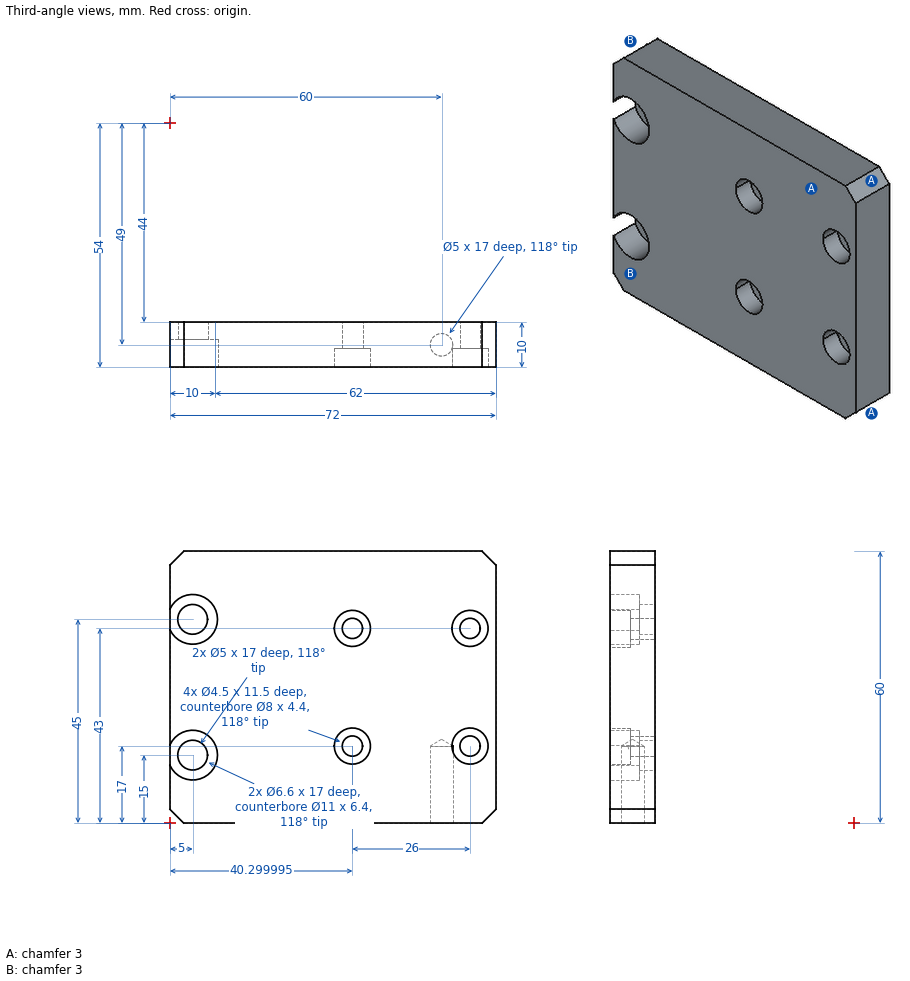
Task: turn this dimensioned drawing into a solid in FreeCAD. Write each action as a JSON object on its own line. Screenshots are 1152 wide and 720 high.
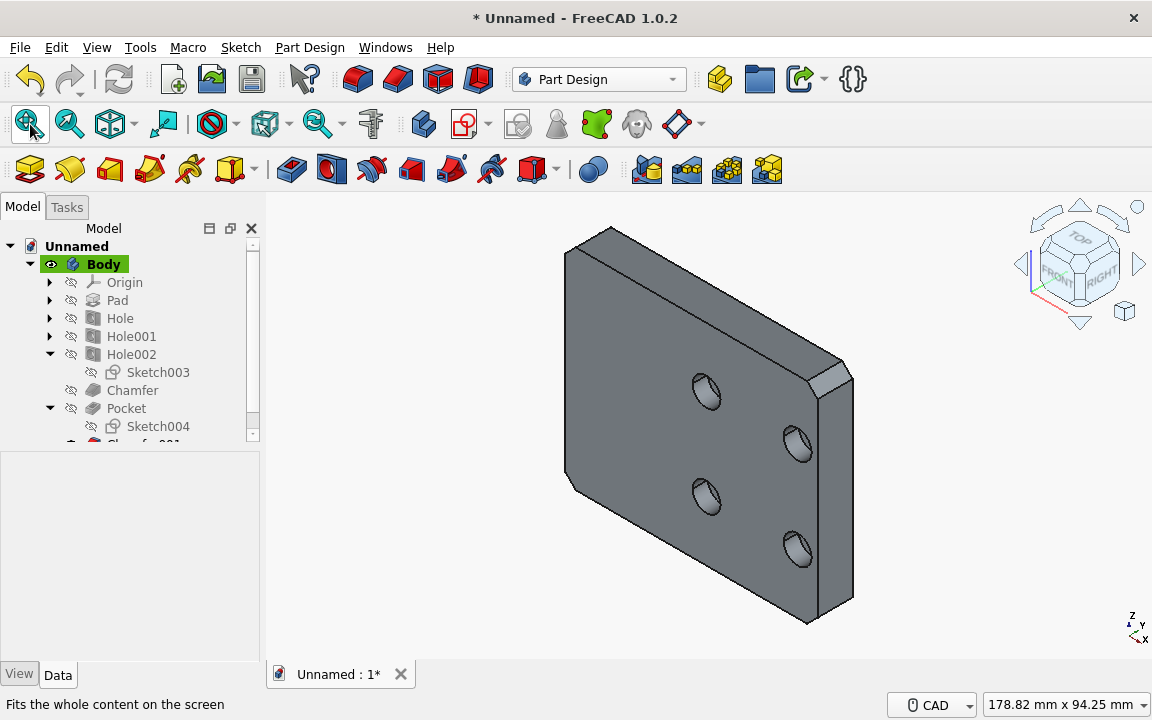
{"action": "left_click", "coordinate": [655, 414]}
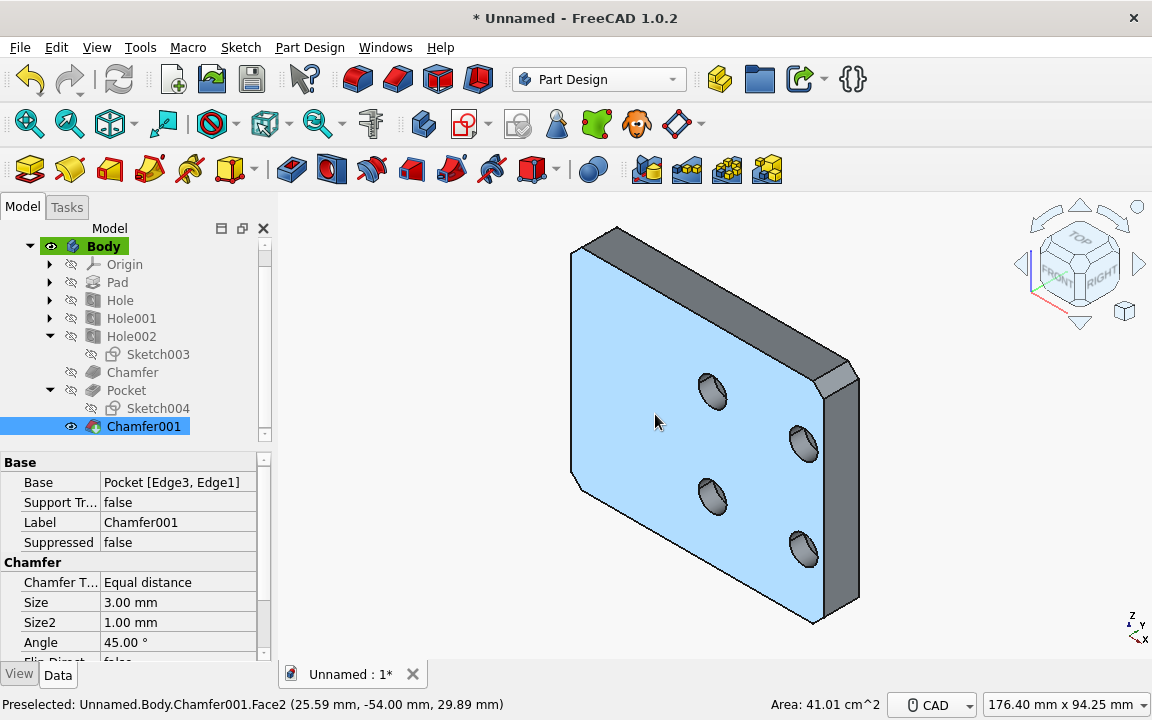
{"action": "left_click", "coordinate": [464, 124]}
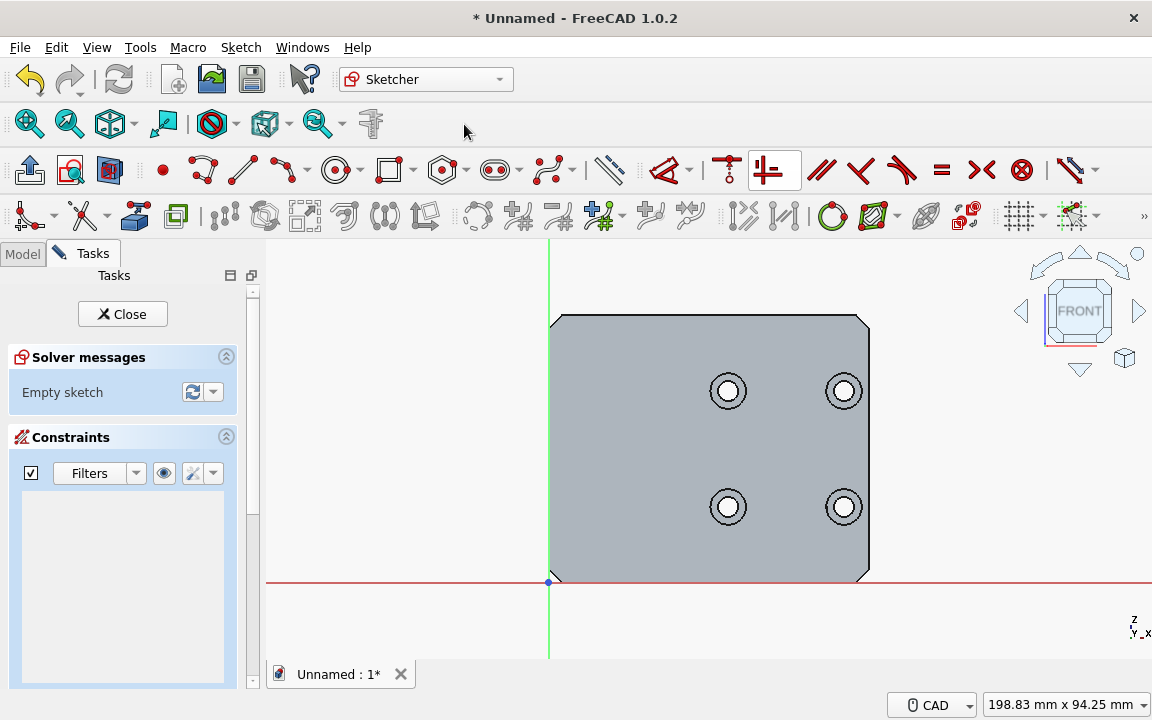
{"action": "left_click", "coordinate": [336, 170]}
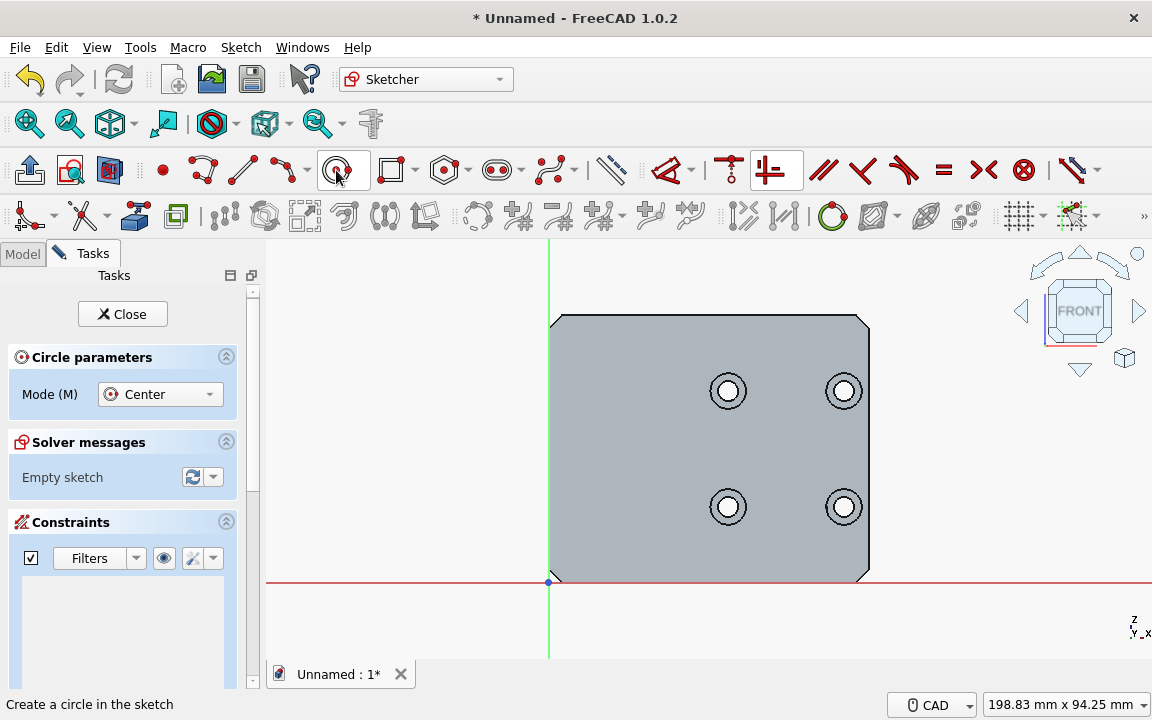
{"action": "scroll", "coordinate": [571, 516], "scroll_direction": "up", "scroll_amount": 3}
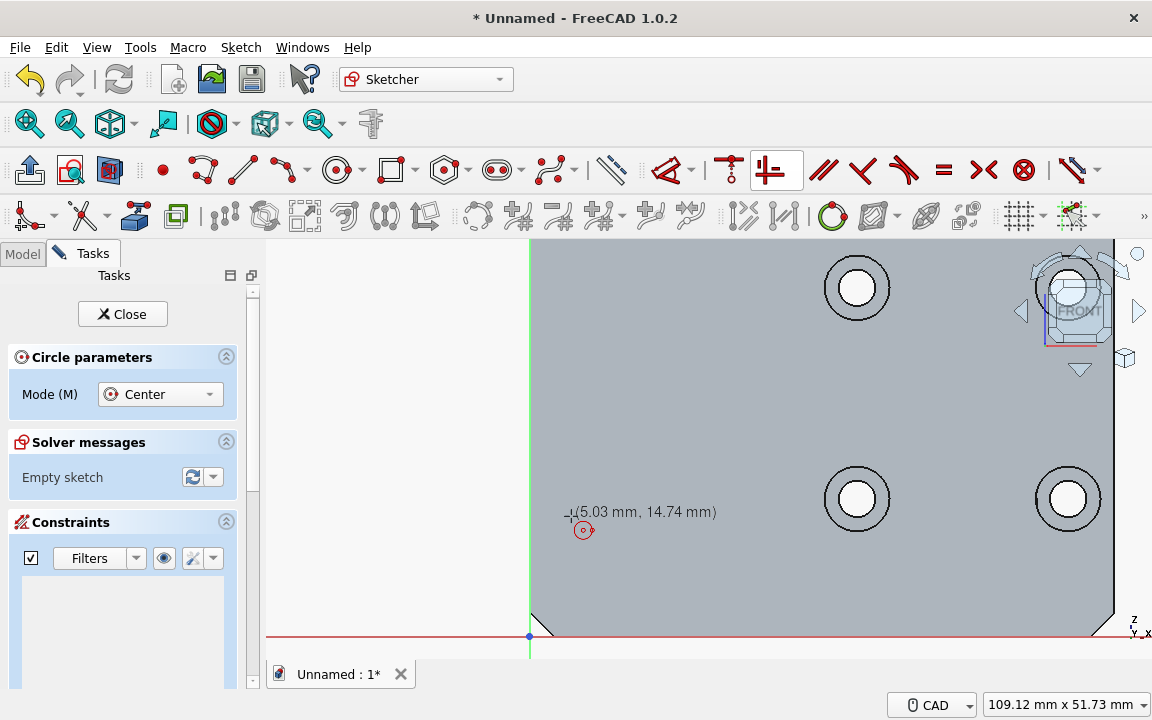
{"action": "left_click", "coordinate": [570, 515]}
{"action": "left_click", "coordinate": [589, 496]}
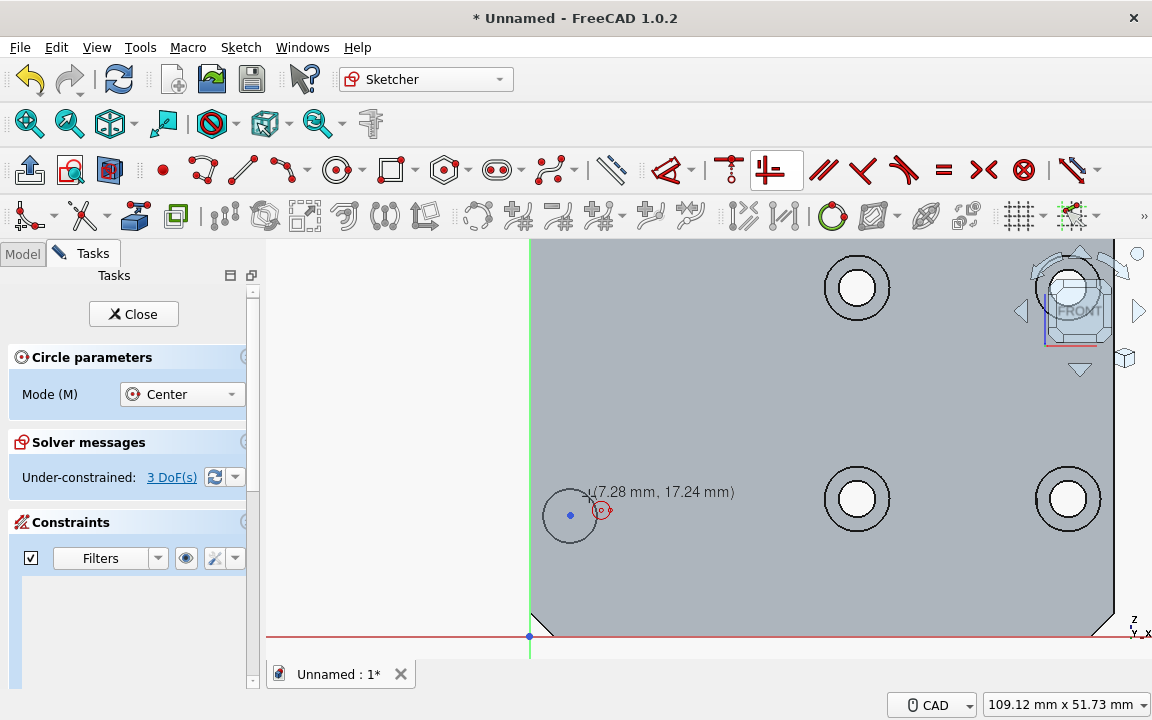
{"action": "left_click", "coordinate": [570, 272]}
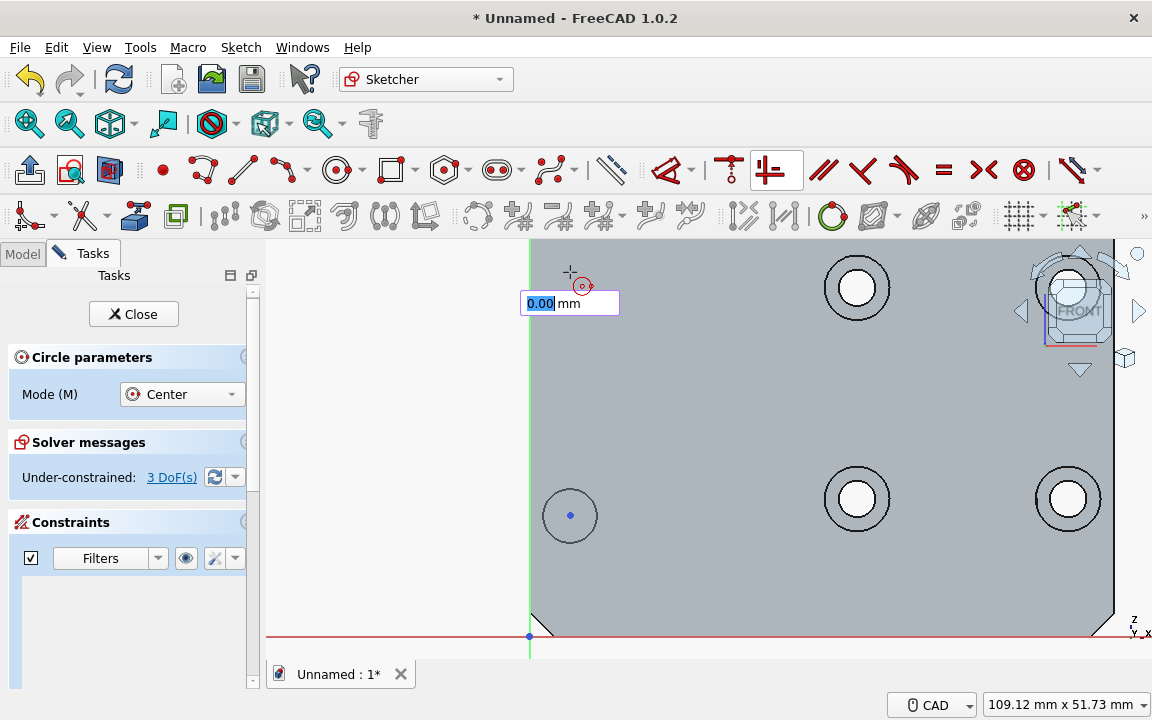
{"action": "scroll", "coordinate": [797, 466], "scroll_direction": "down", "scroll_amount": 2}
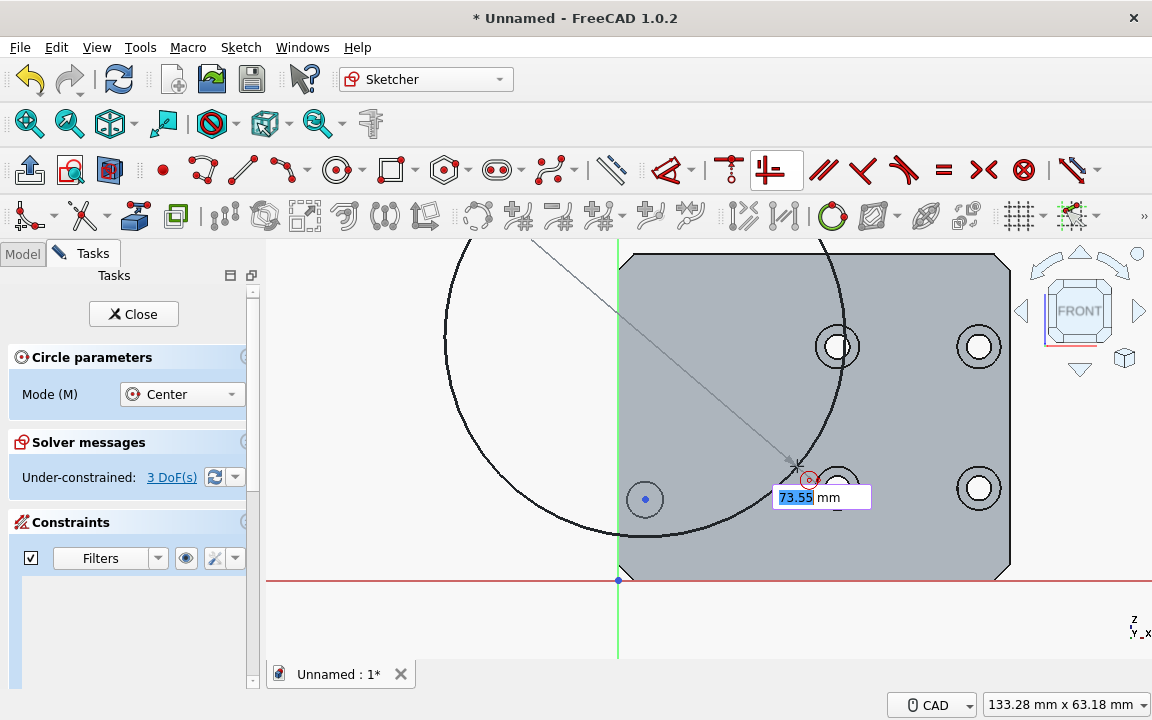
{"action": "left_click", "coordinate": [658, 323]}
{"action": "key", "text": "Escape"}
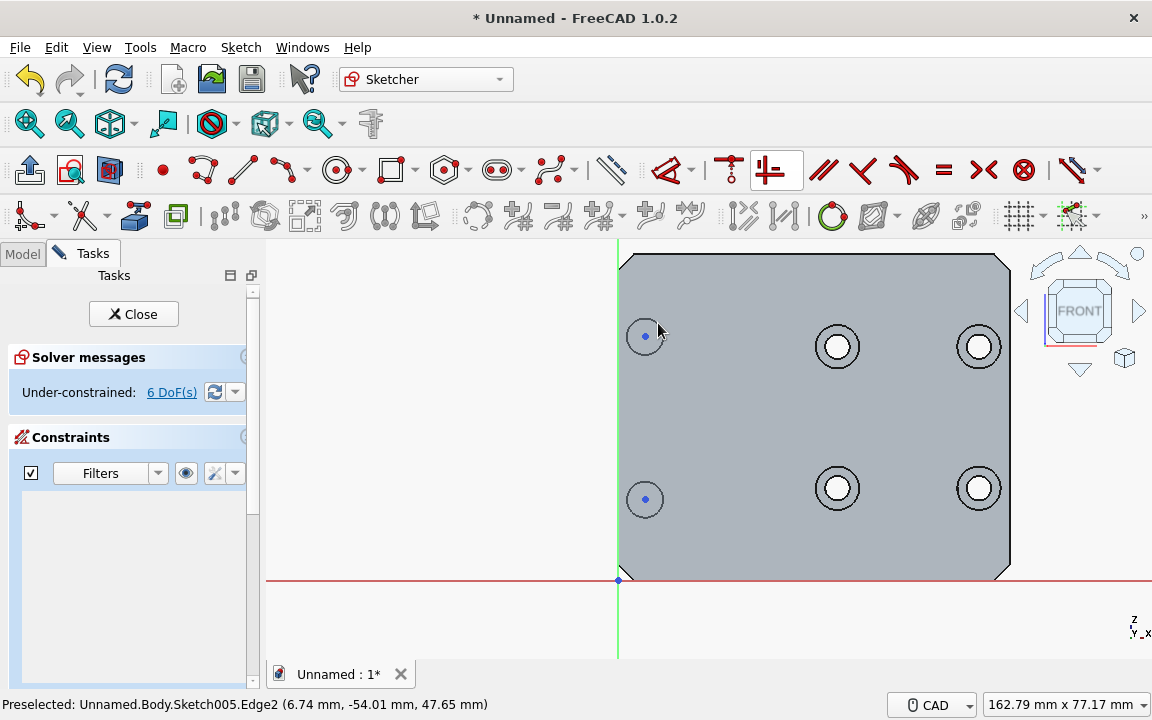
{"action": "left_click", "coordinate": [658, 487]}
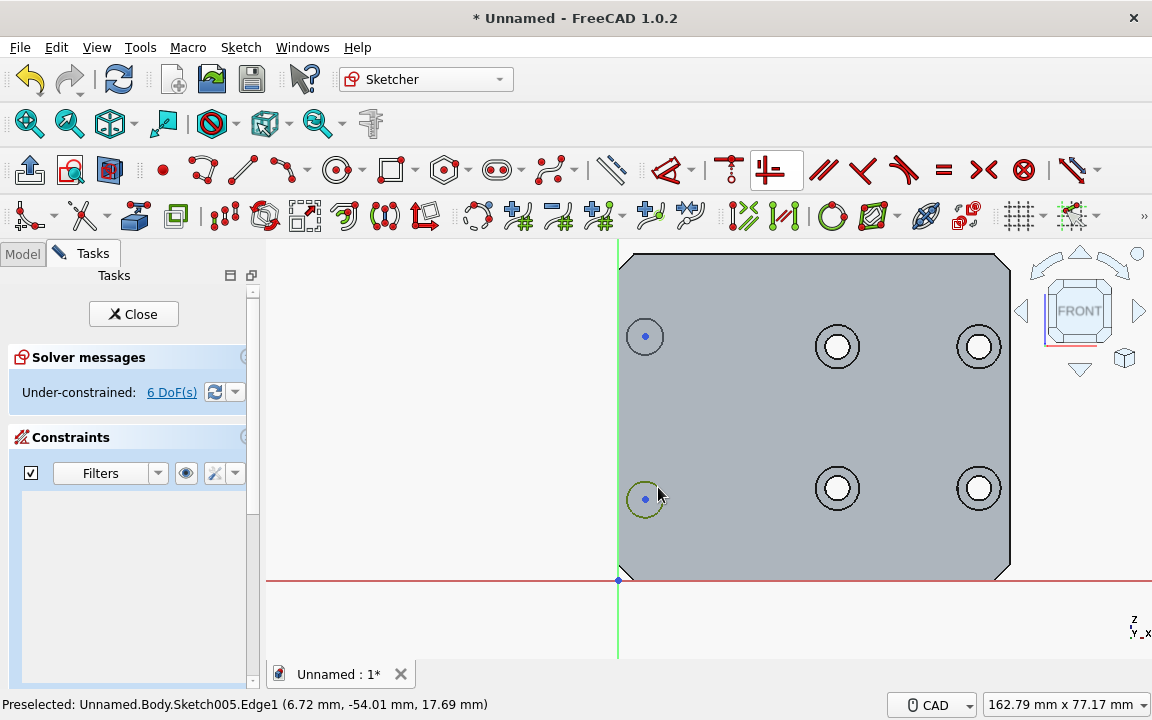
{"action": "left_click", "coordinate": [658, 324]}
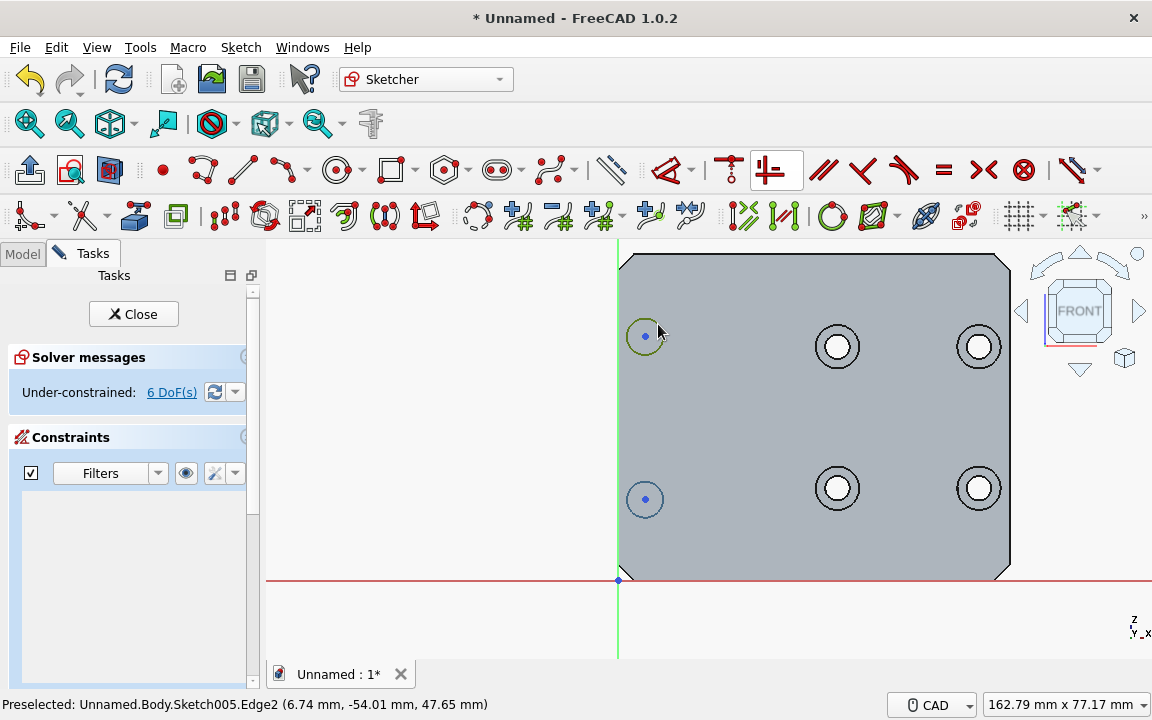
{"action": "left_click", "coordinate": [944, 170]}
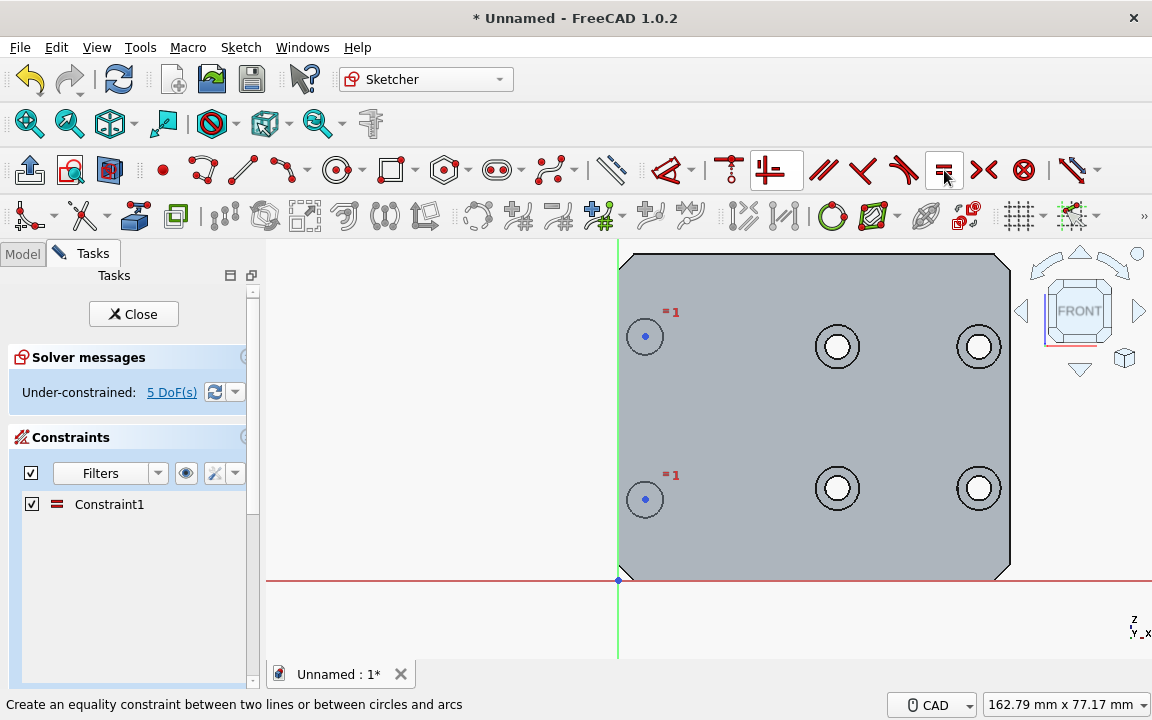
{"action": "left_click", "coordinate": [645, 500]}